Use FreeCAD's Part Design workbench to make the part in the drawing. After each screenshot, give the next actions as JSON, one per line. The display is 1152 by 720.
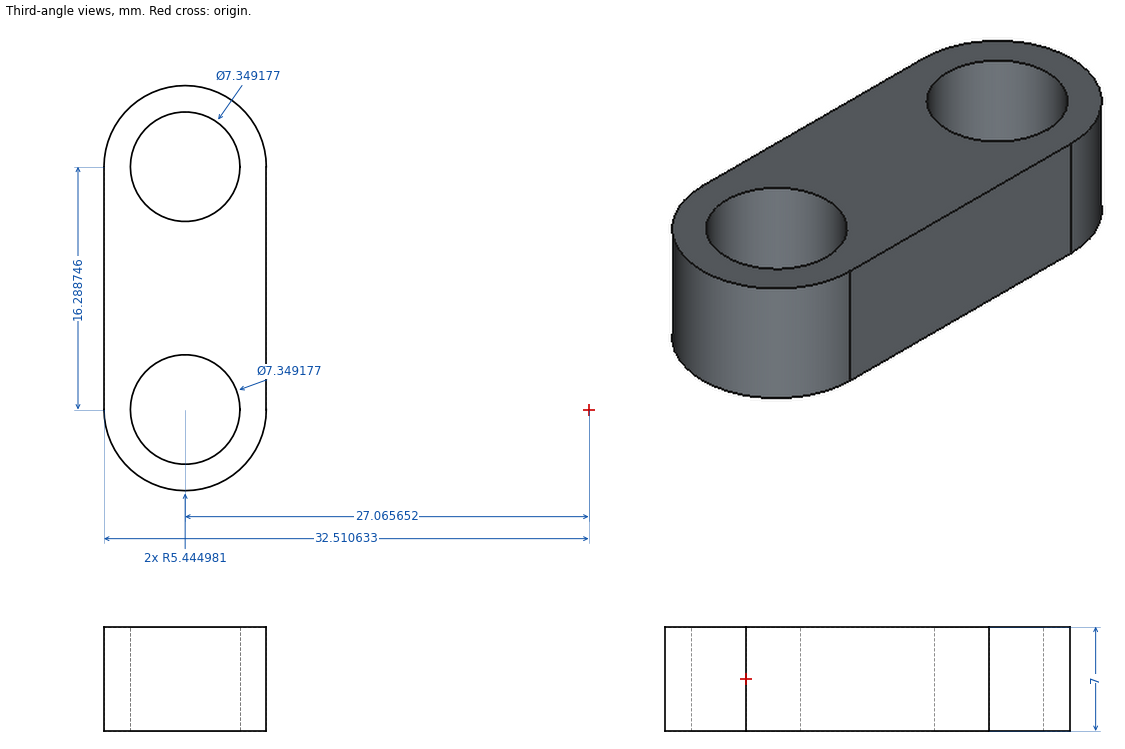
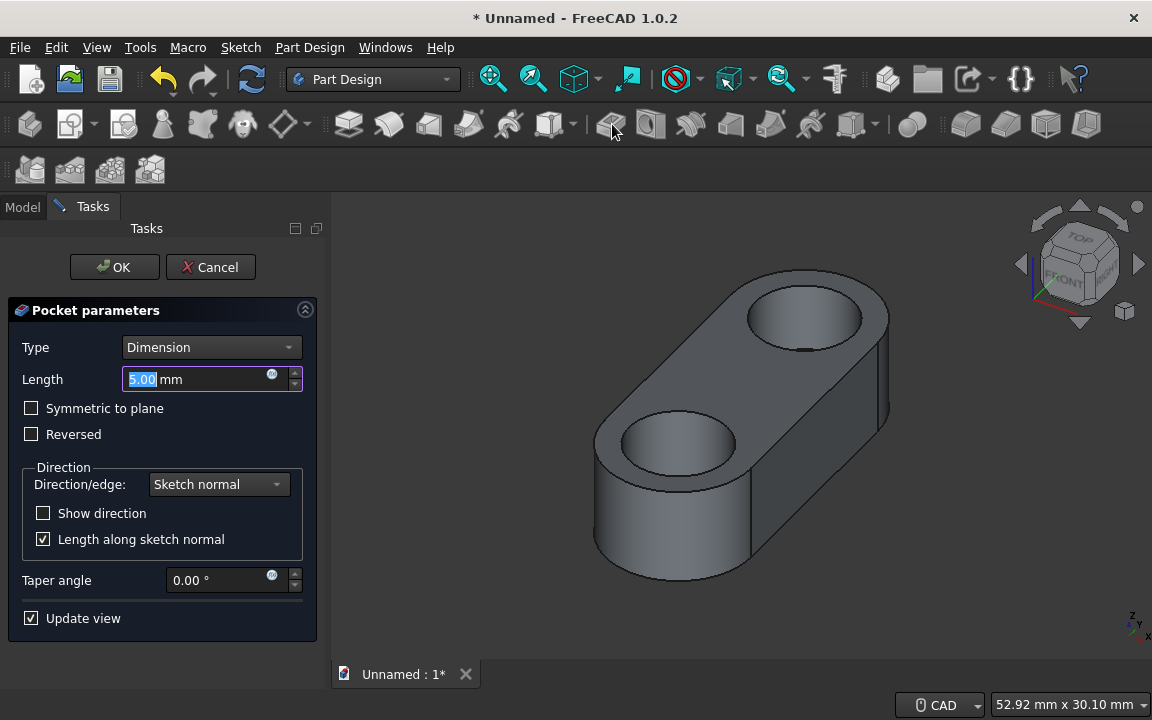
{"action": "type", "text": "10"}
{"action": "key", "text": "Tab"}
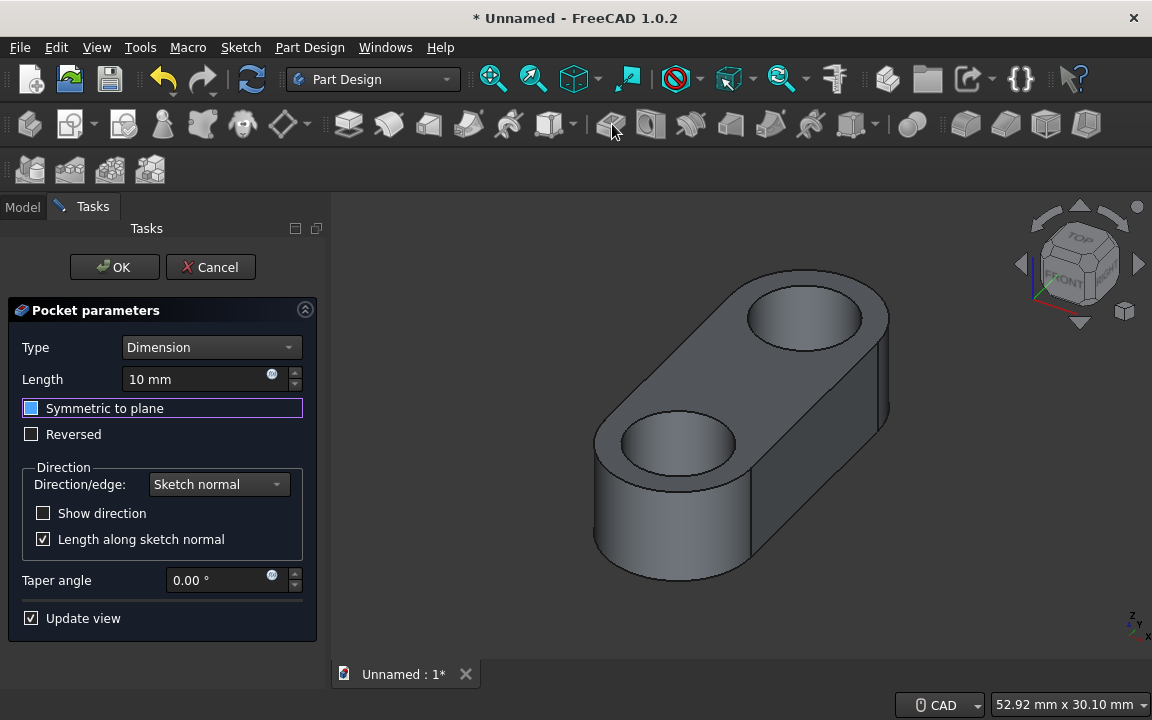
{"action": "left_click", "coordinate": [115, 267]}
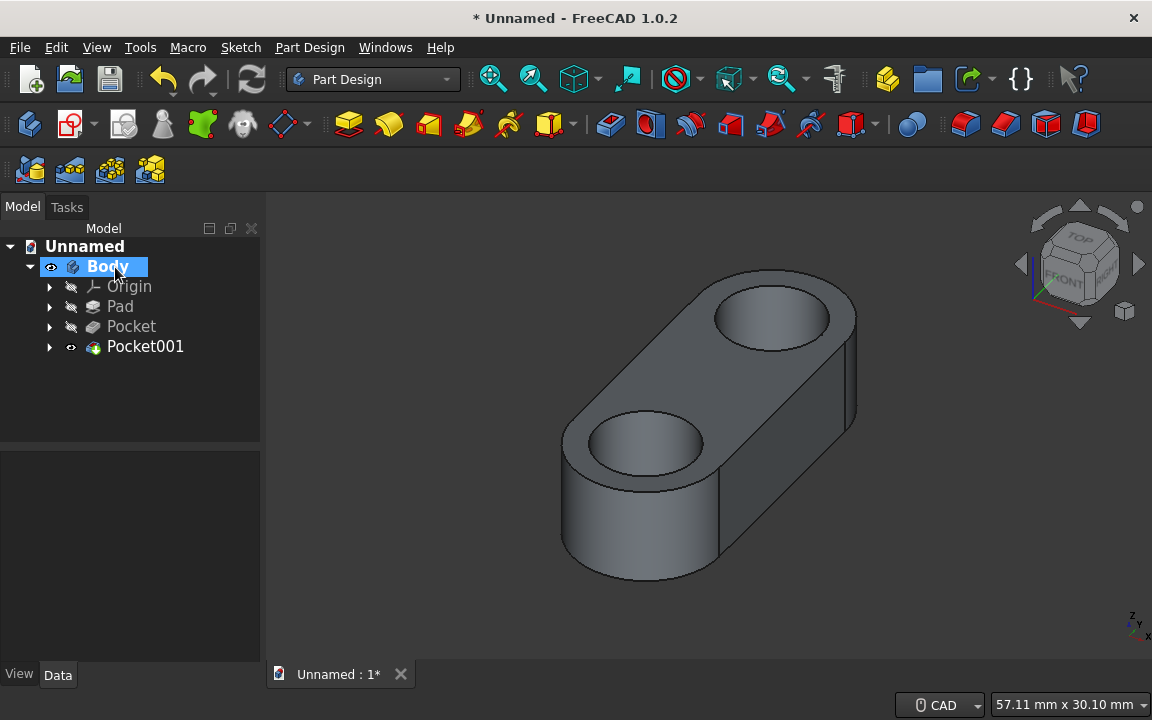
{"action": "key", "text": "0"}